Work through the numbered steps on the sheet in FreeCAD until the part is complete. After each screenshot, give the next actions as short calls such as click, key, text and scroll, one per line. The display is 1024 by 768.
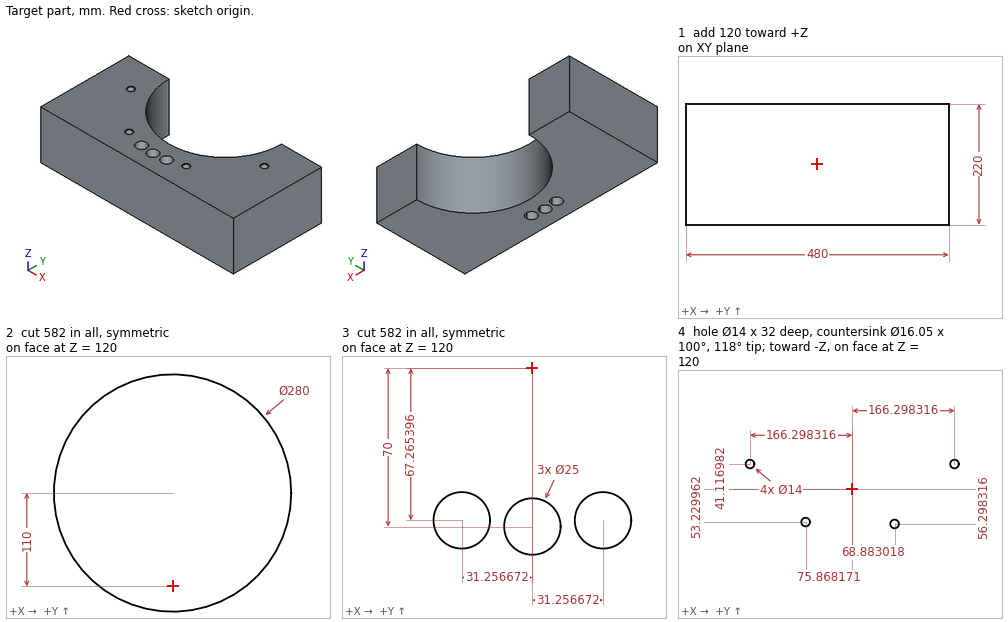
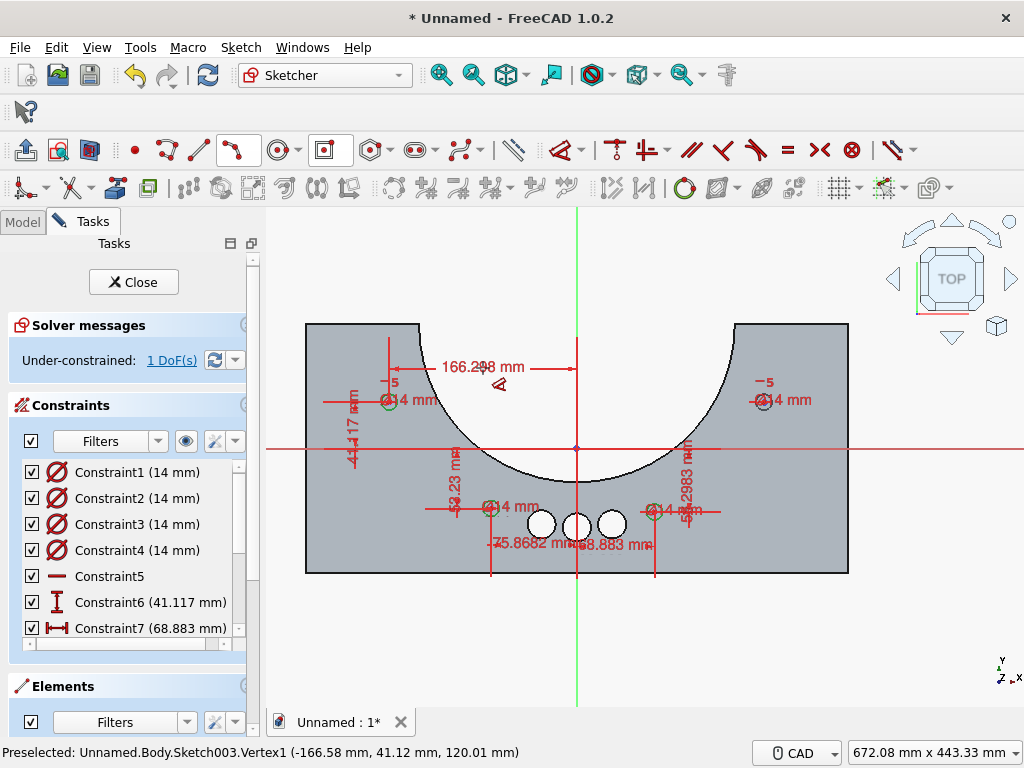
click(764, 402)
click(670, 368)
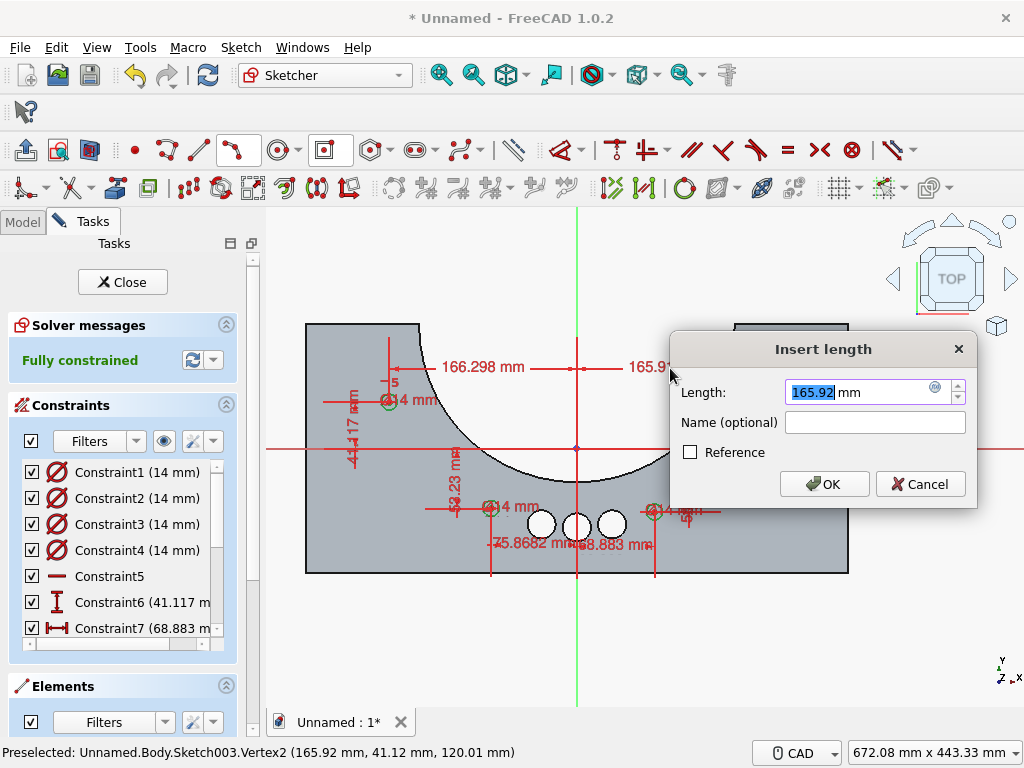
text(166.298316)
key(Return)
key(Escape)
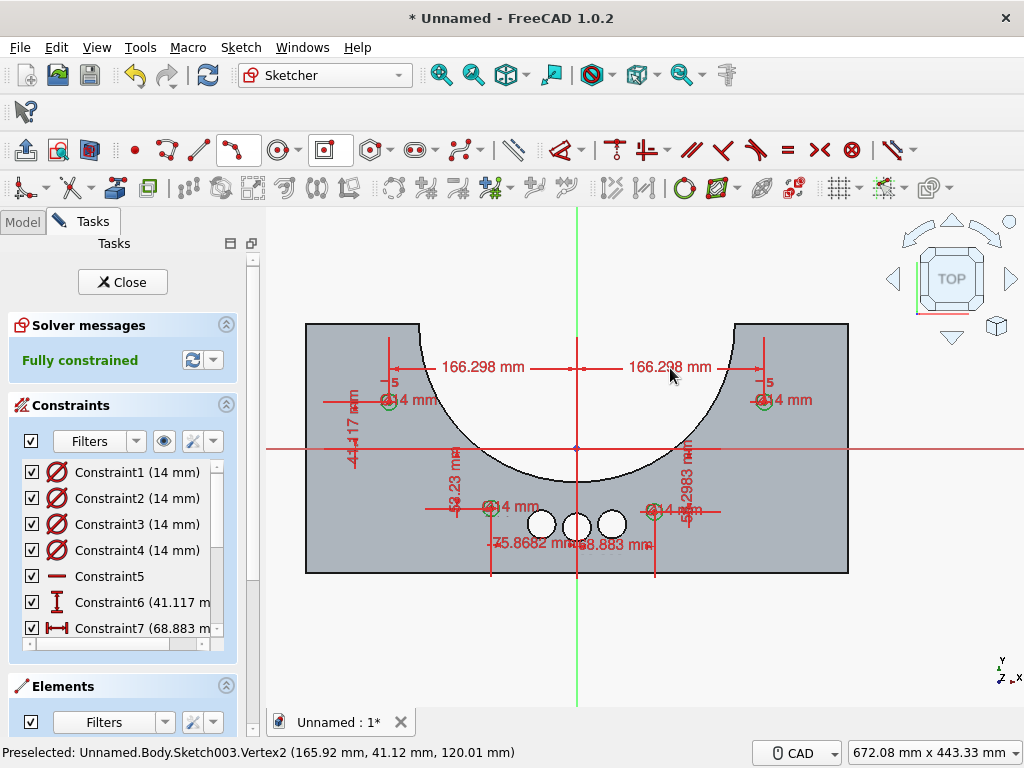
click(123, 282)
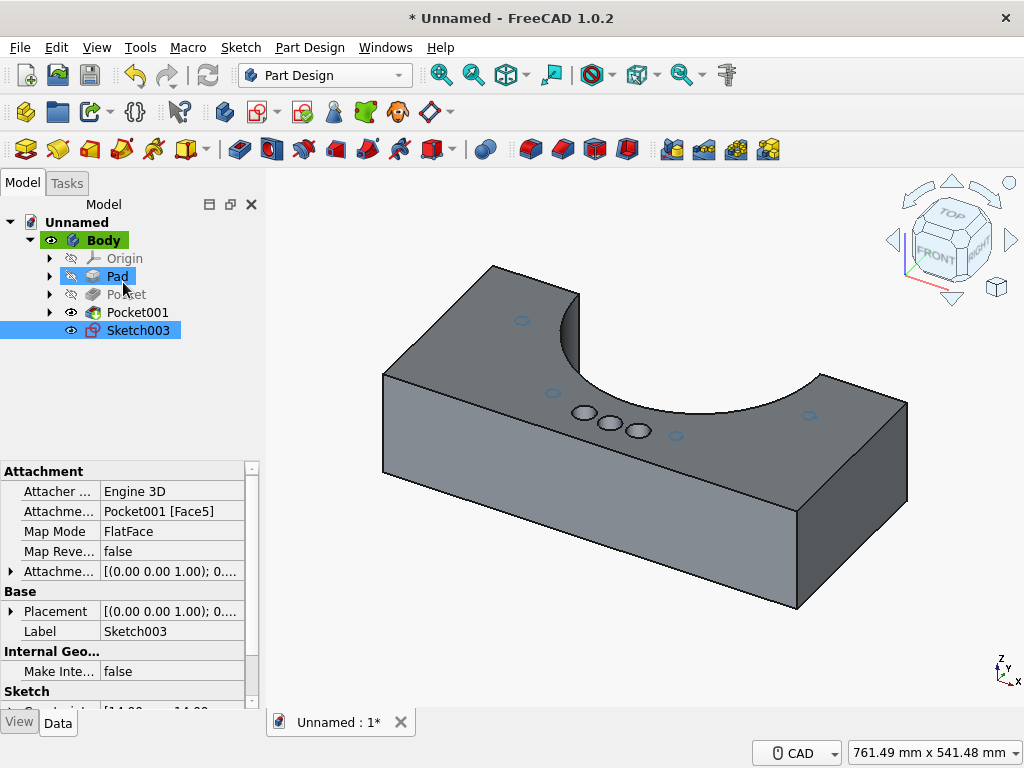
click(272, 150)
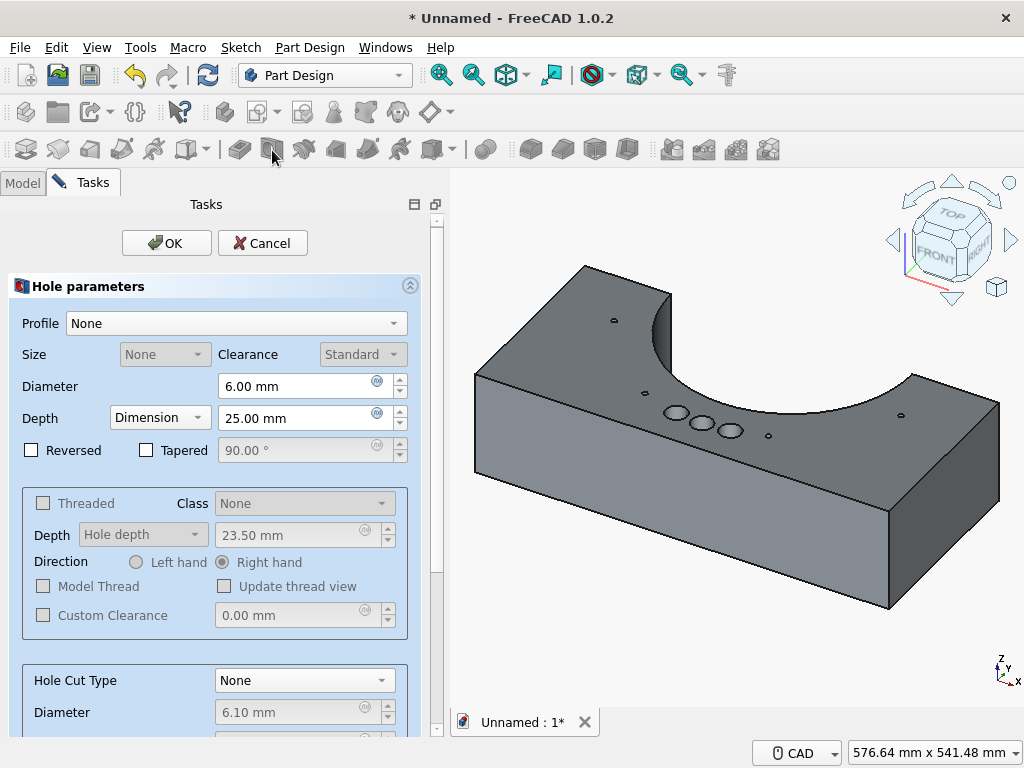
triple_click(305, 386)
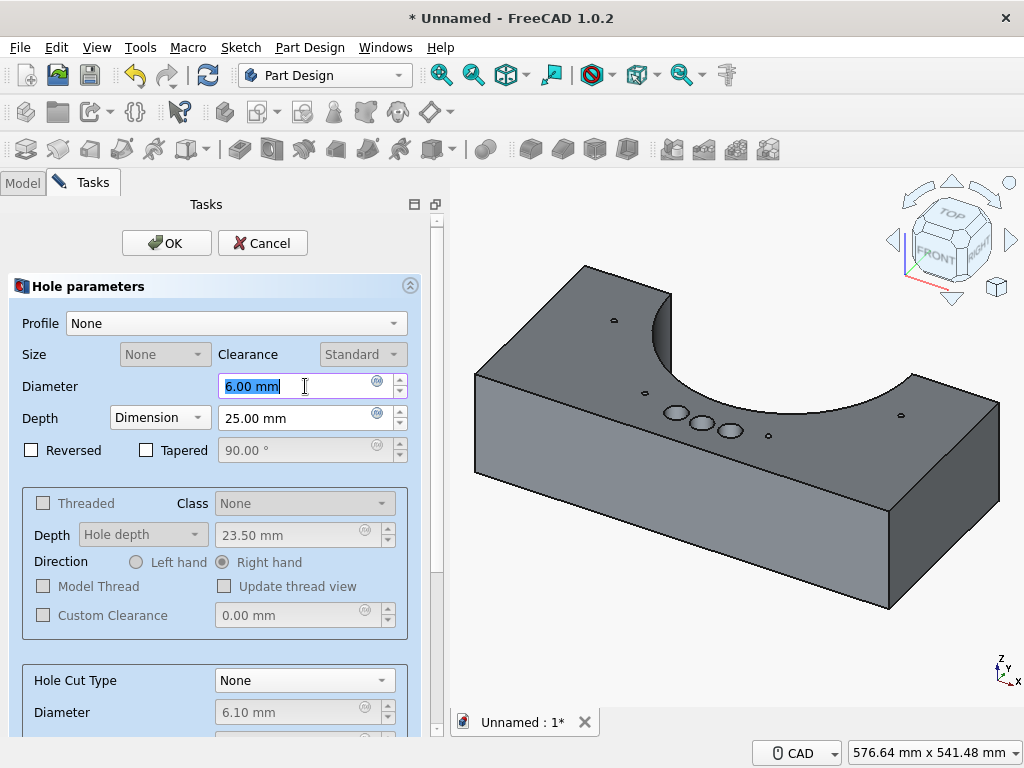
text(14)
key(Tab)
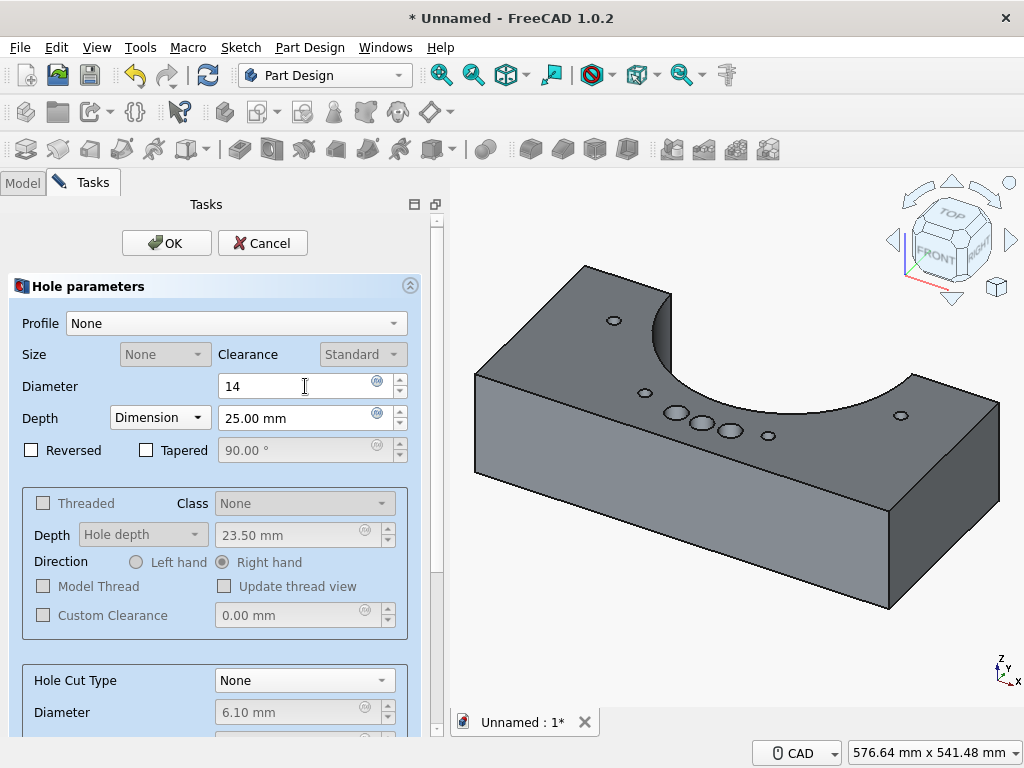
triple_click(305, 418)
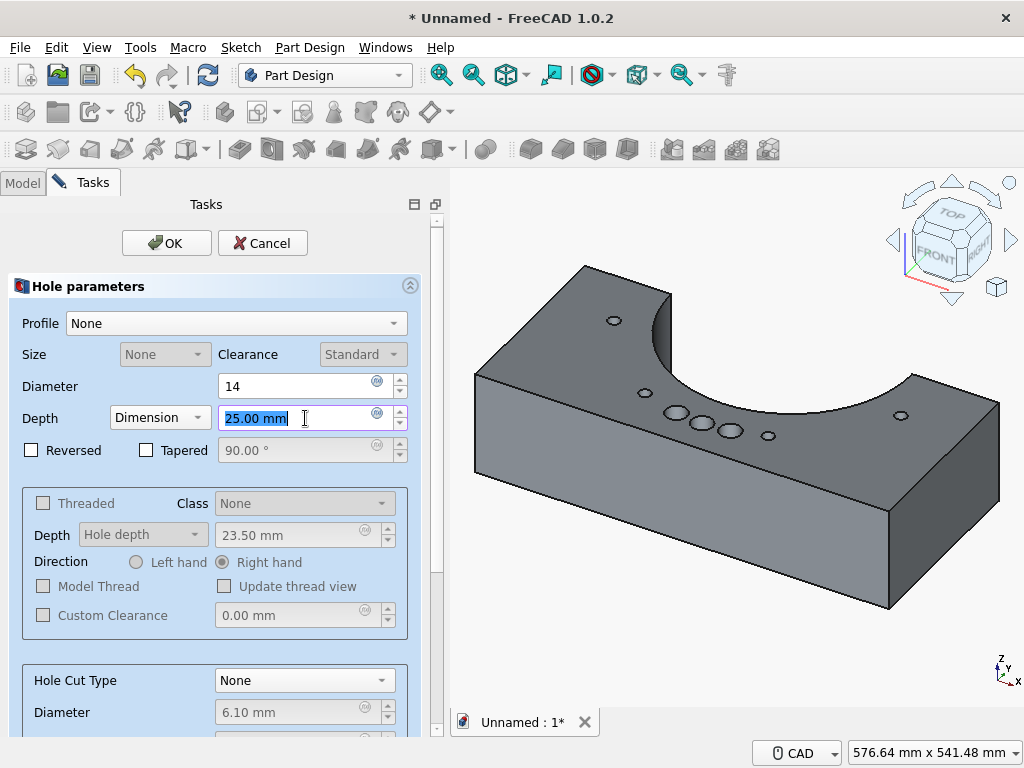
text(32)
key(Tab)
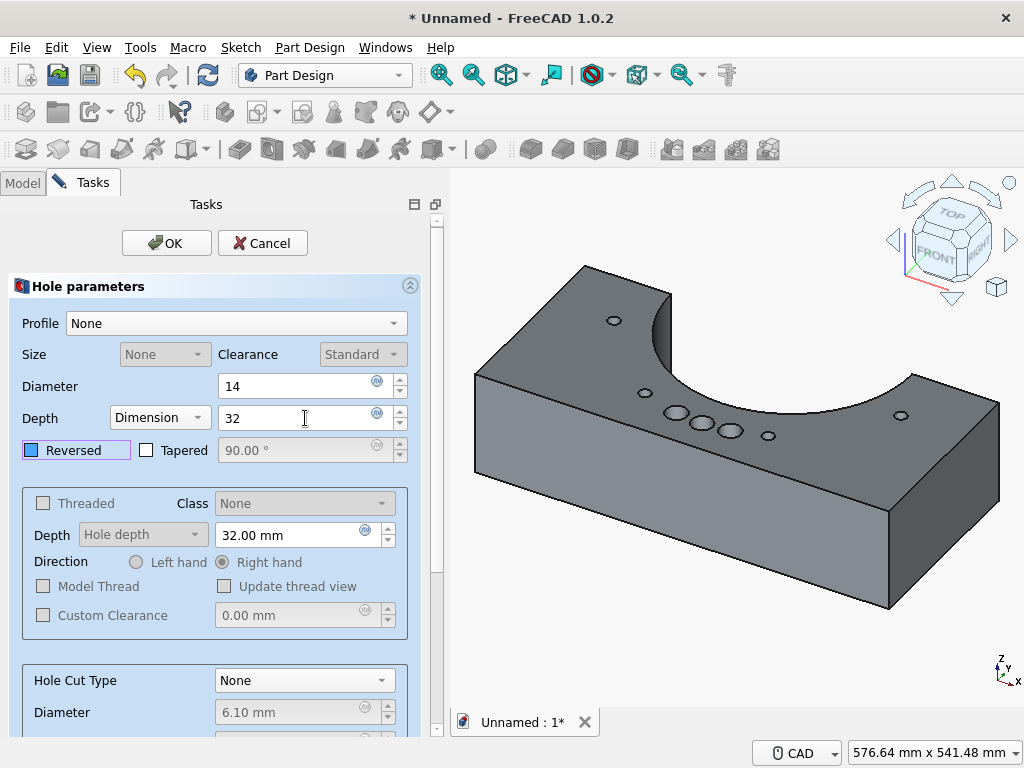
click(306, 680)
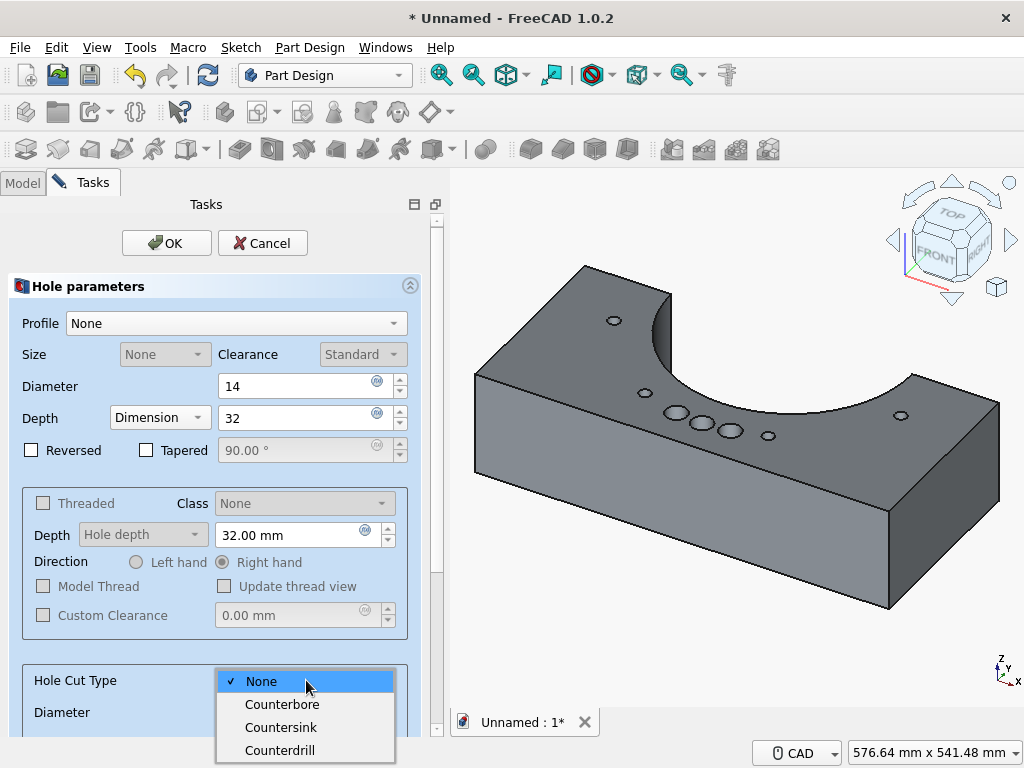
click(304, 728)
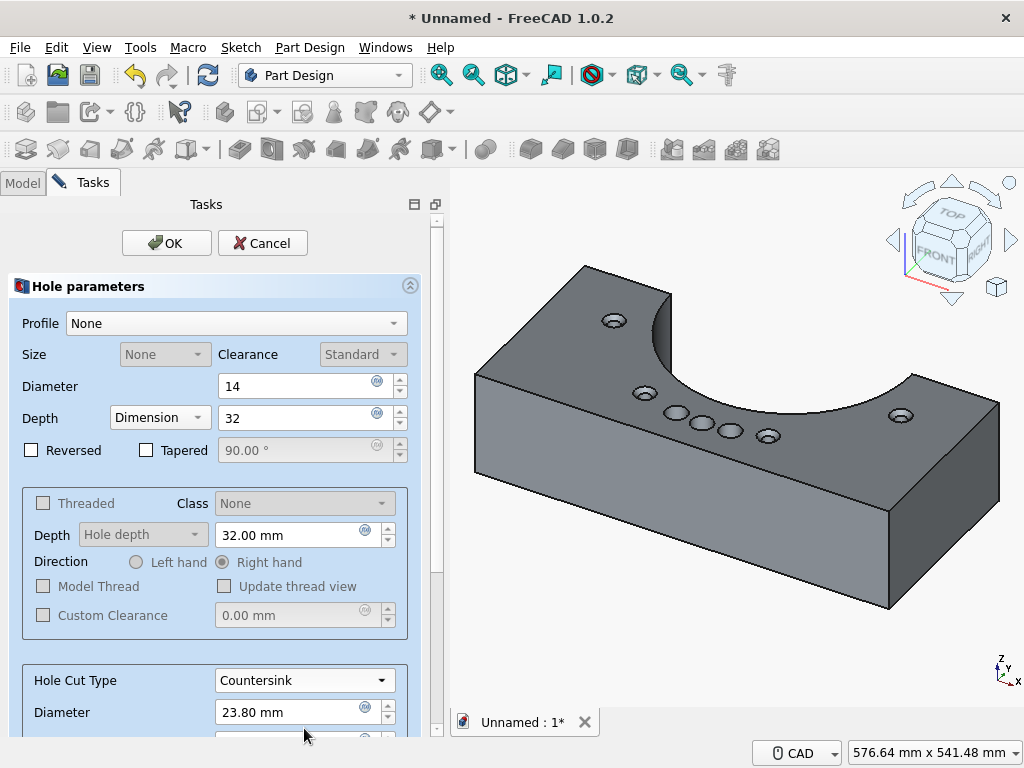
scroll(437, 475, down, 2)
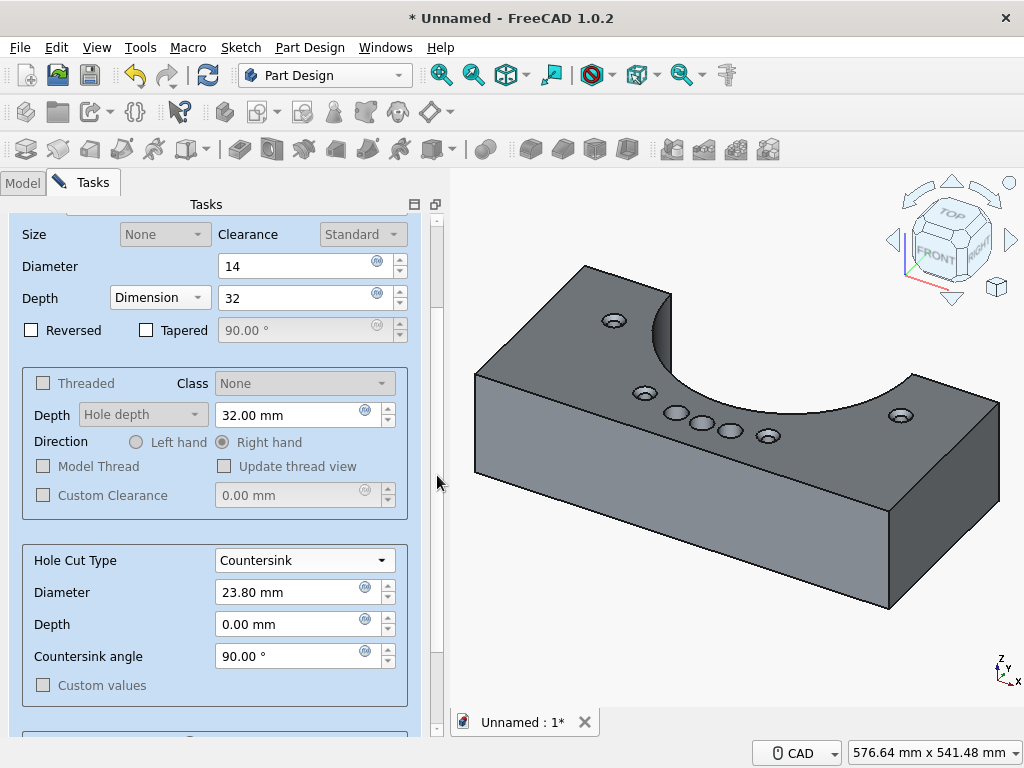
triple_click(298, 656)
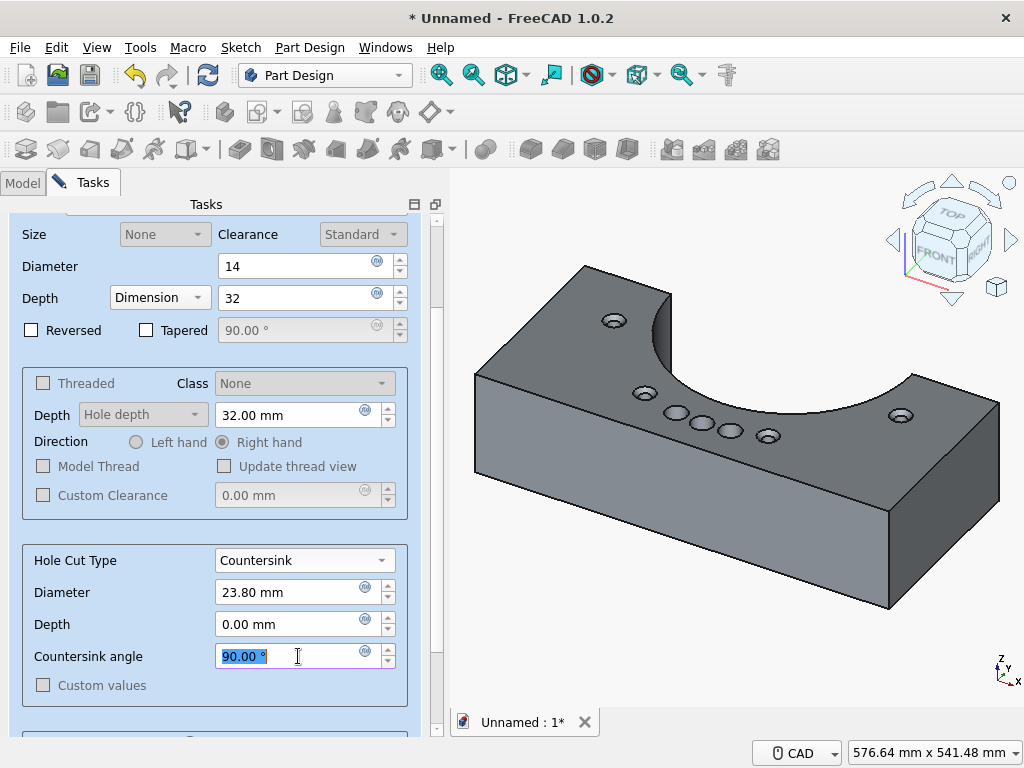
text(100)
key(Tab)